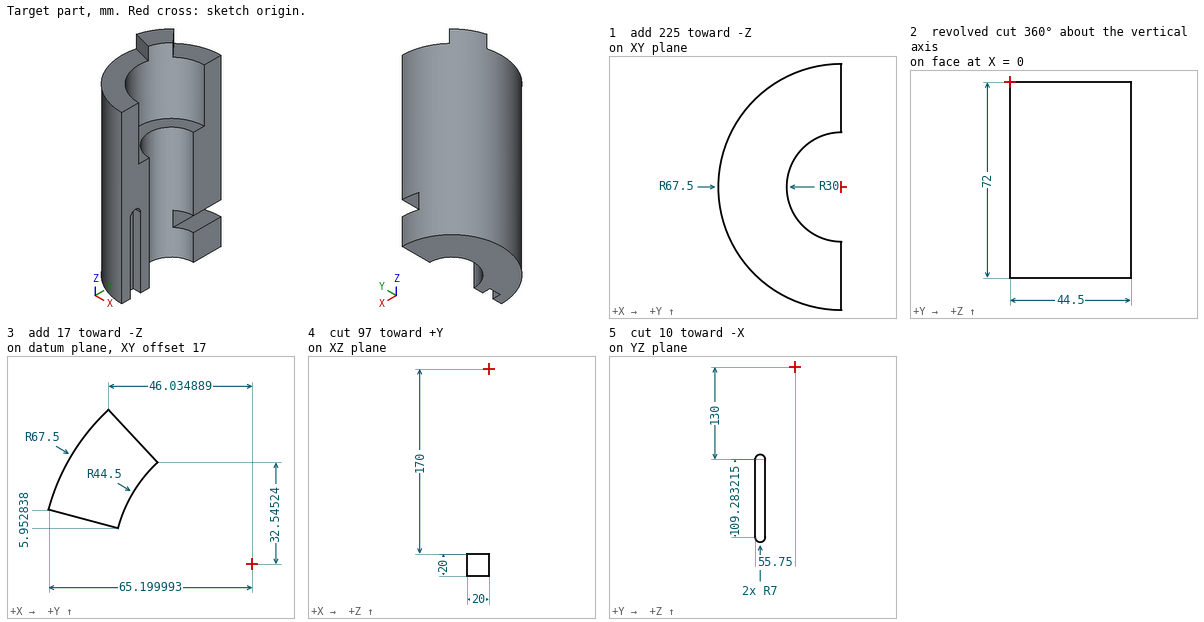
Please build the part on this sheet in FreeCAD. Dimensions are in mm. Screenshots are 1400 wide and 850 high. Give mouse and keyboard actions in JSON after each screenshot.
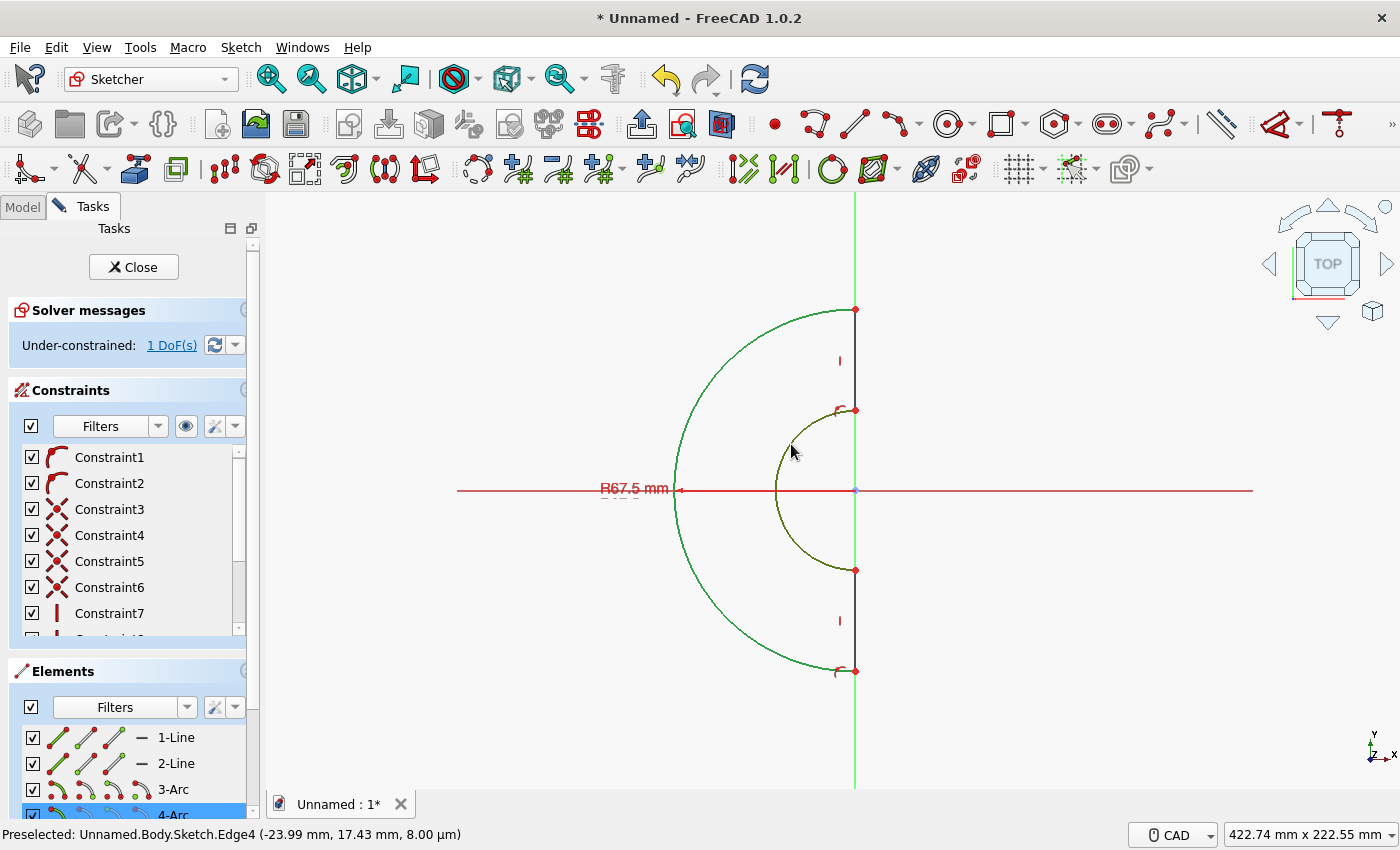
{"action": "key", "text": "k r"}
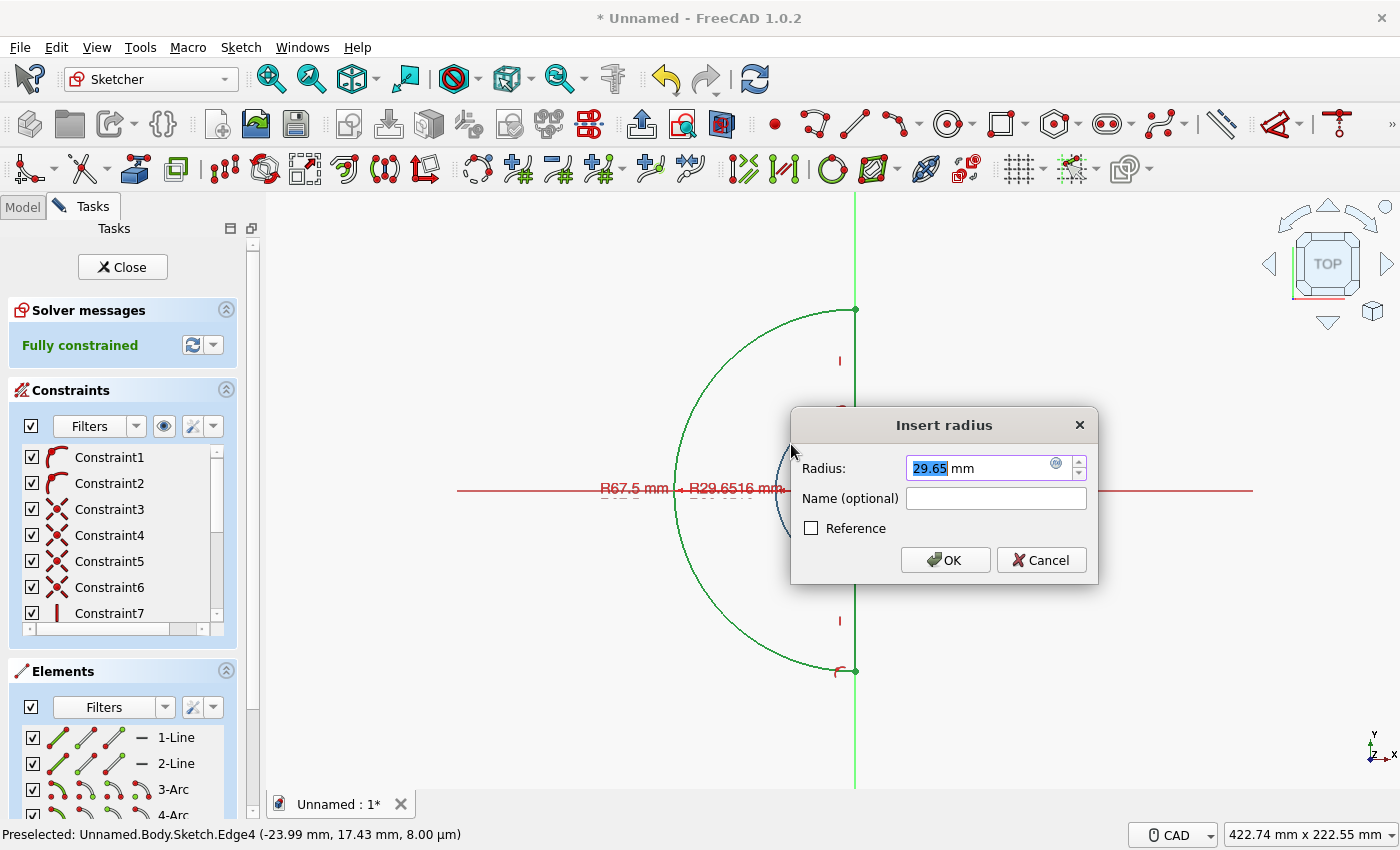
{"action": "type", "text": "30"}
{"action": "key", "text": "Return"}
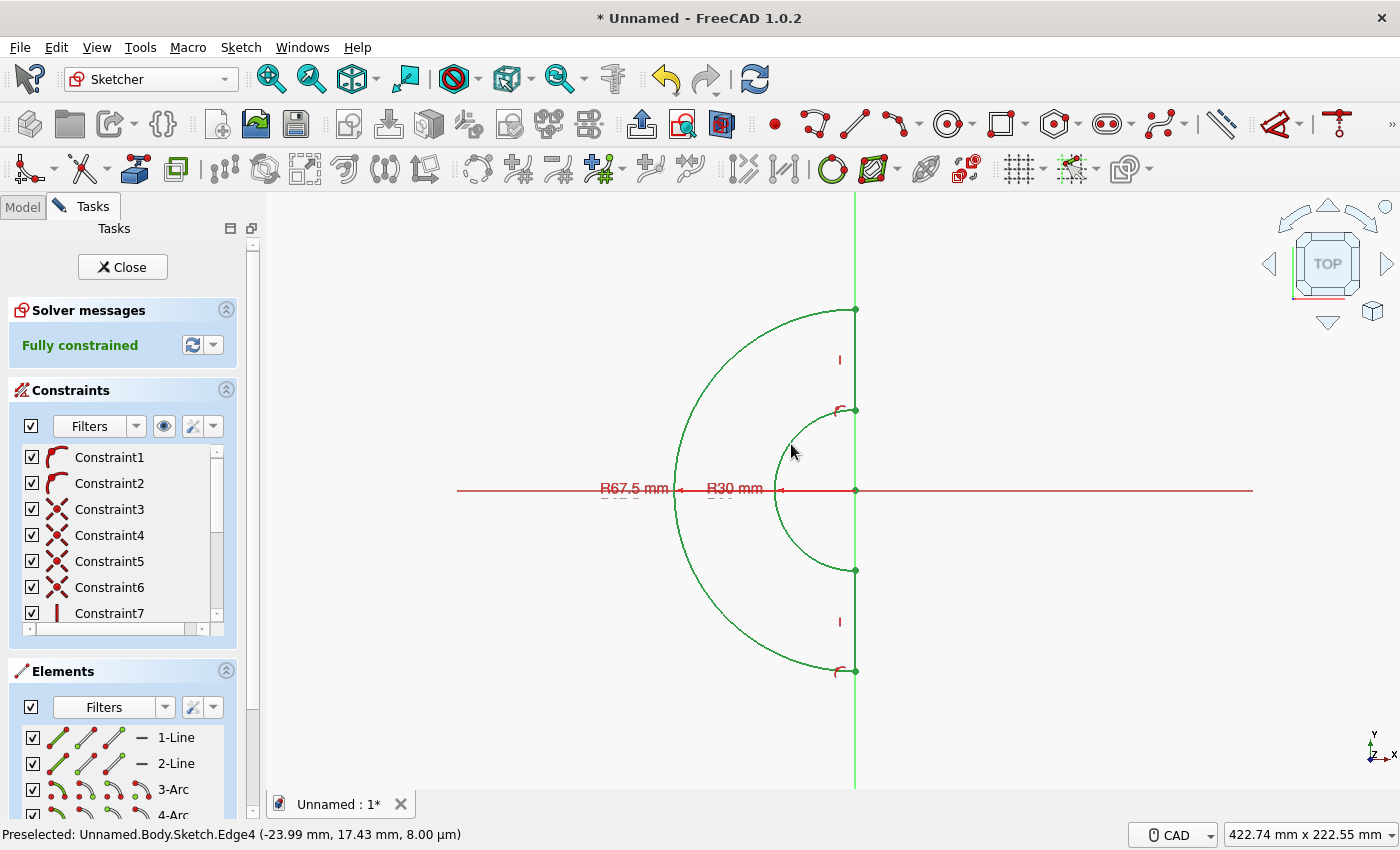
{"action": "left_click", "coordinate": [123, 267]}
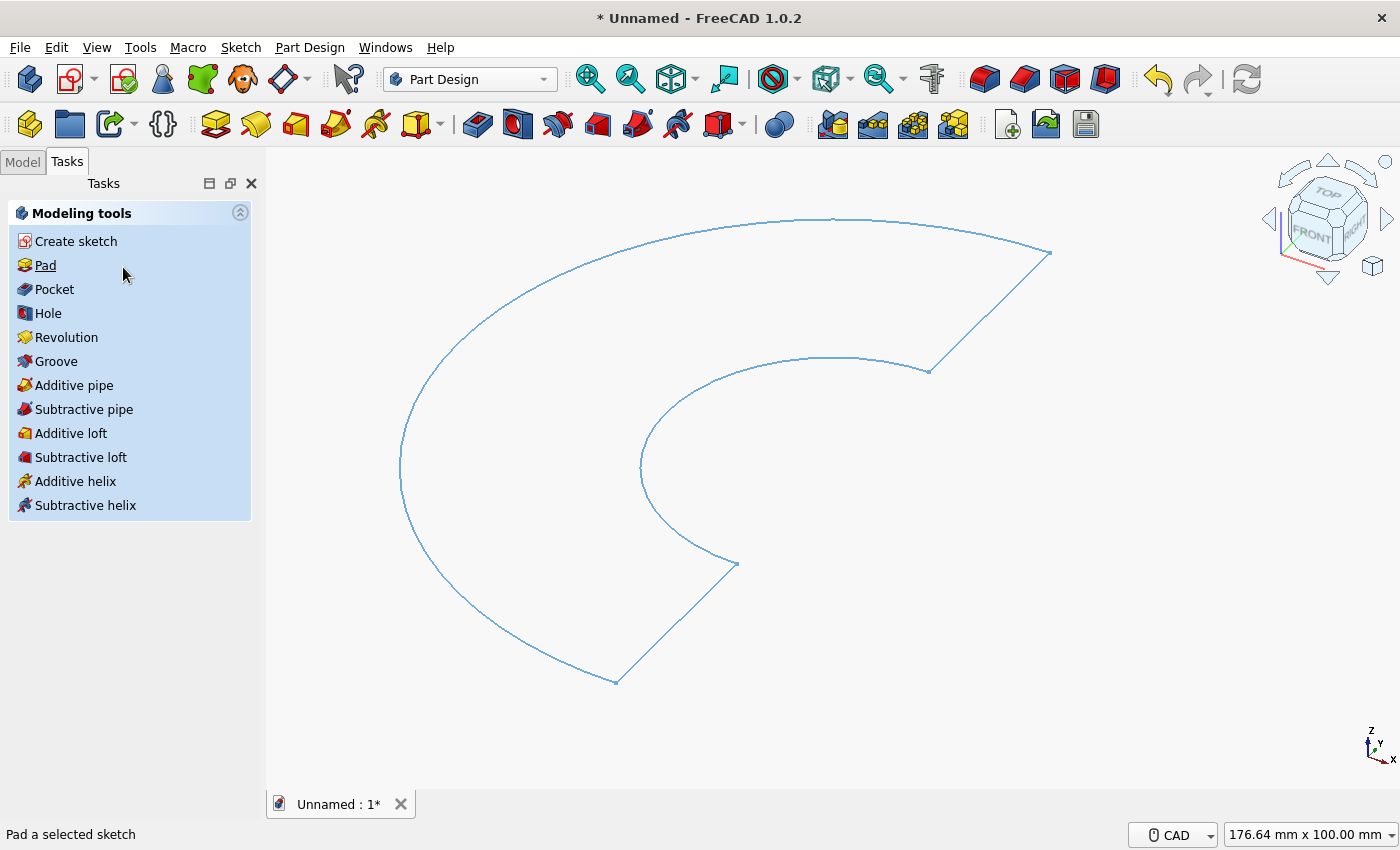
{"action": "left_click", "coordinate": [216, 124]}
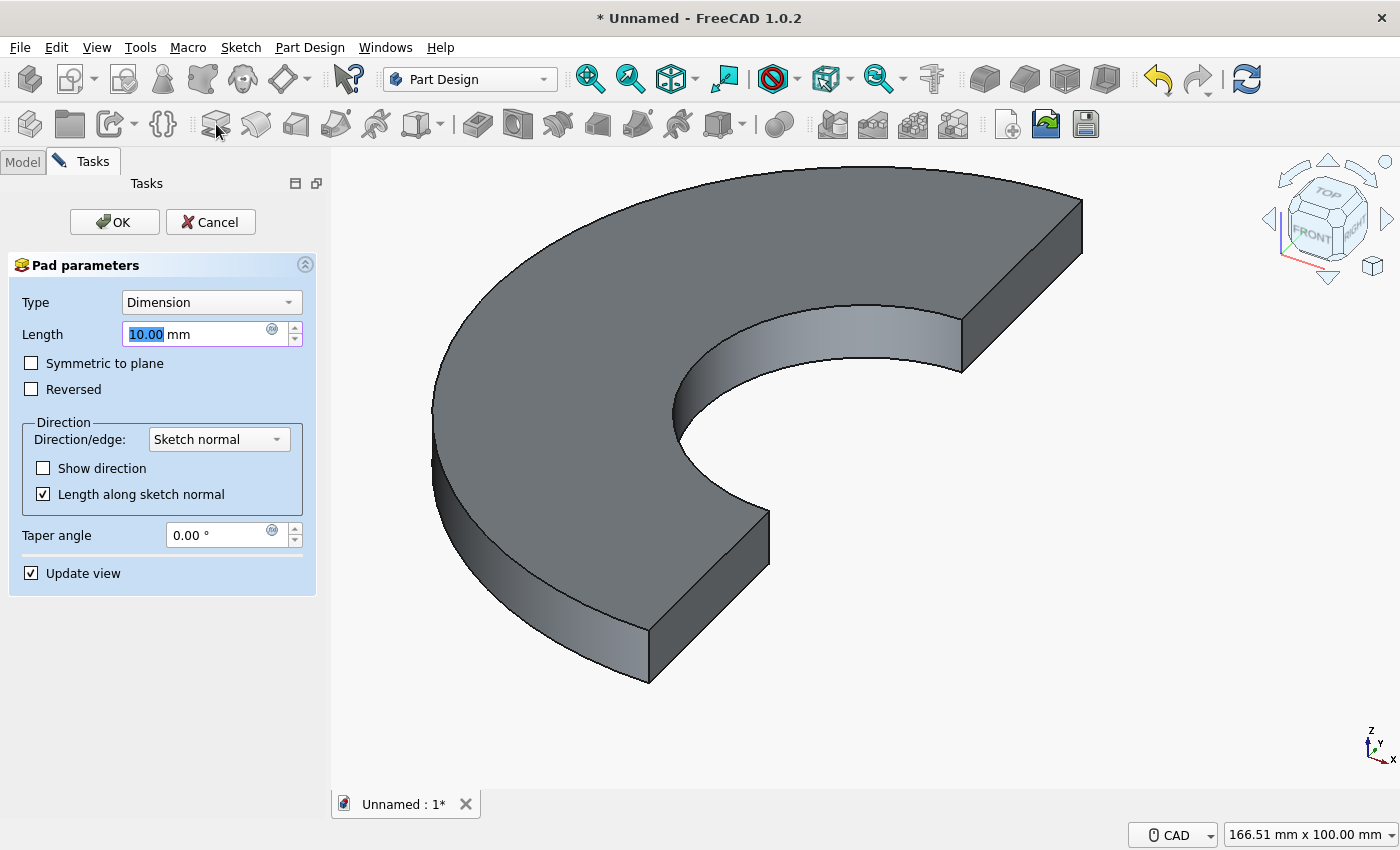
{"action": "type", "text": "225"}
{"action": "key", "text": "Tab"}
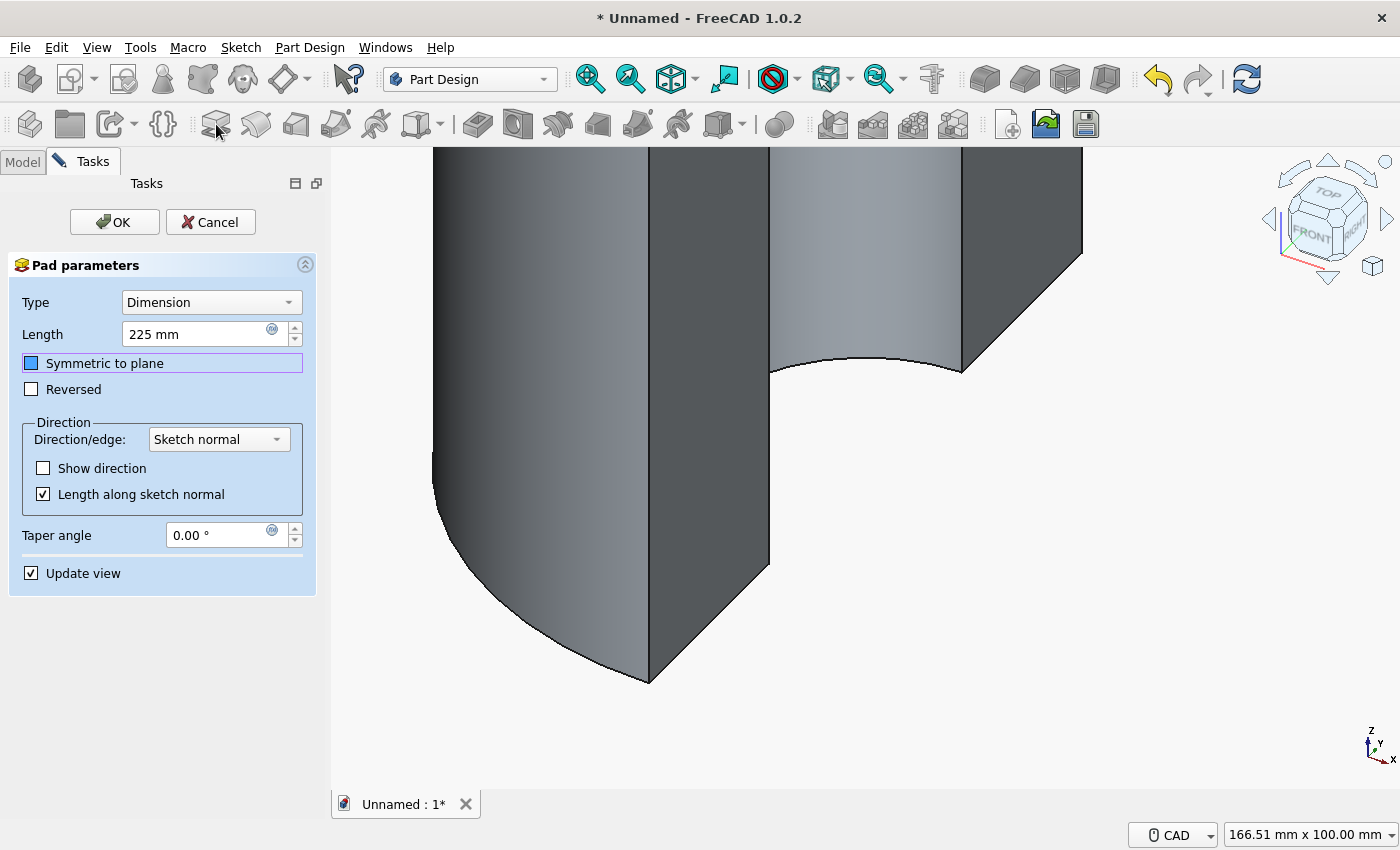
{"action": "left_click", "coordinate": [30, 389]}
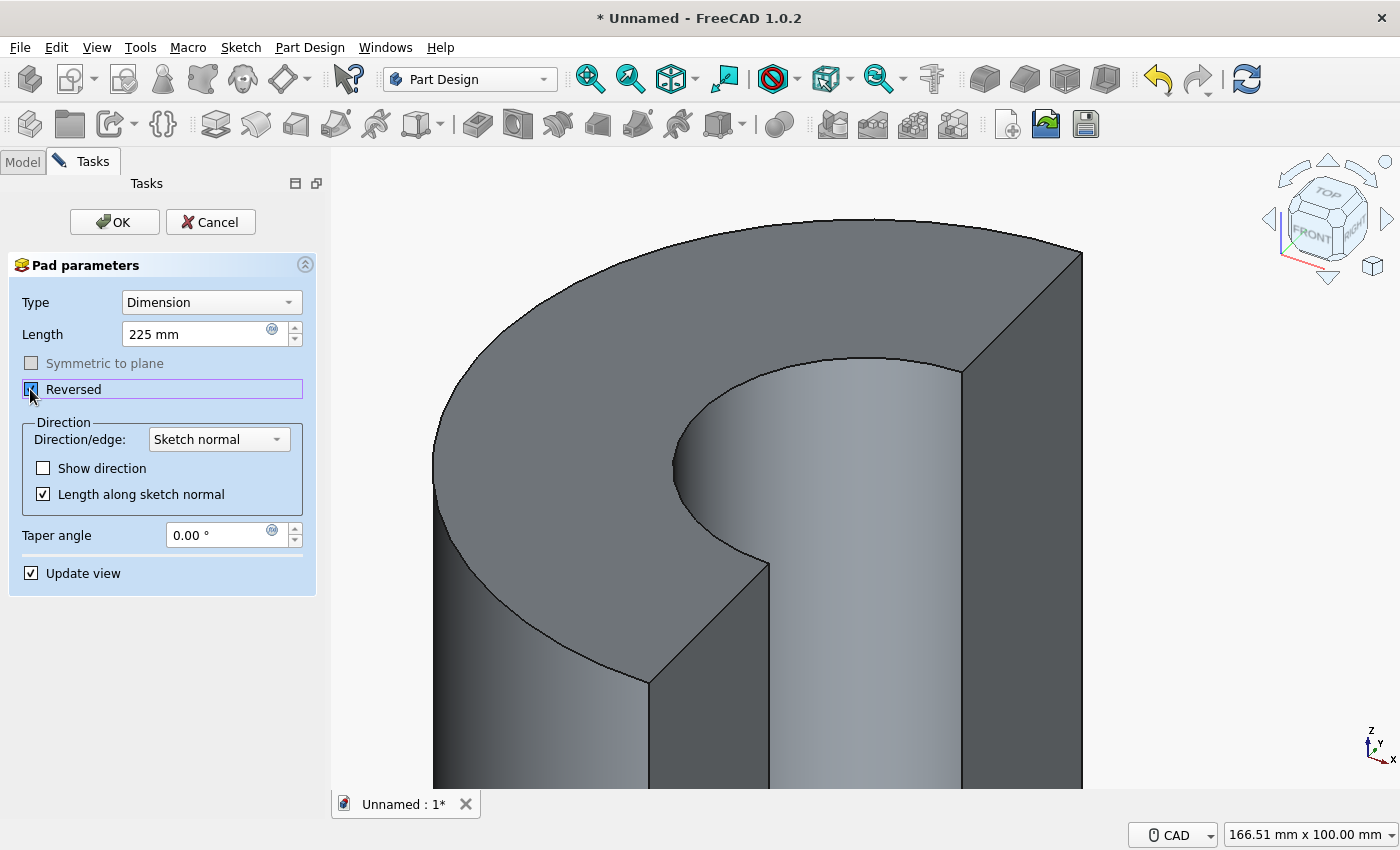
{"action": "left_click", "coordinate": [115, 222]}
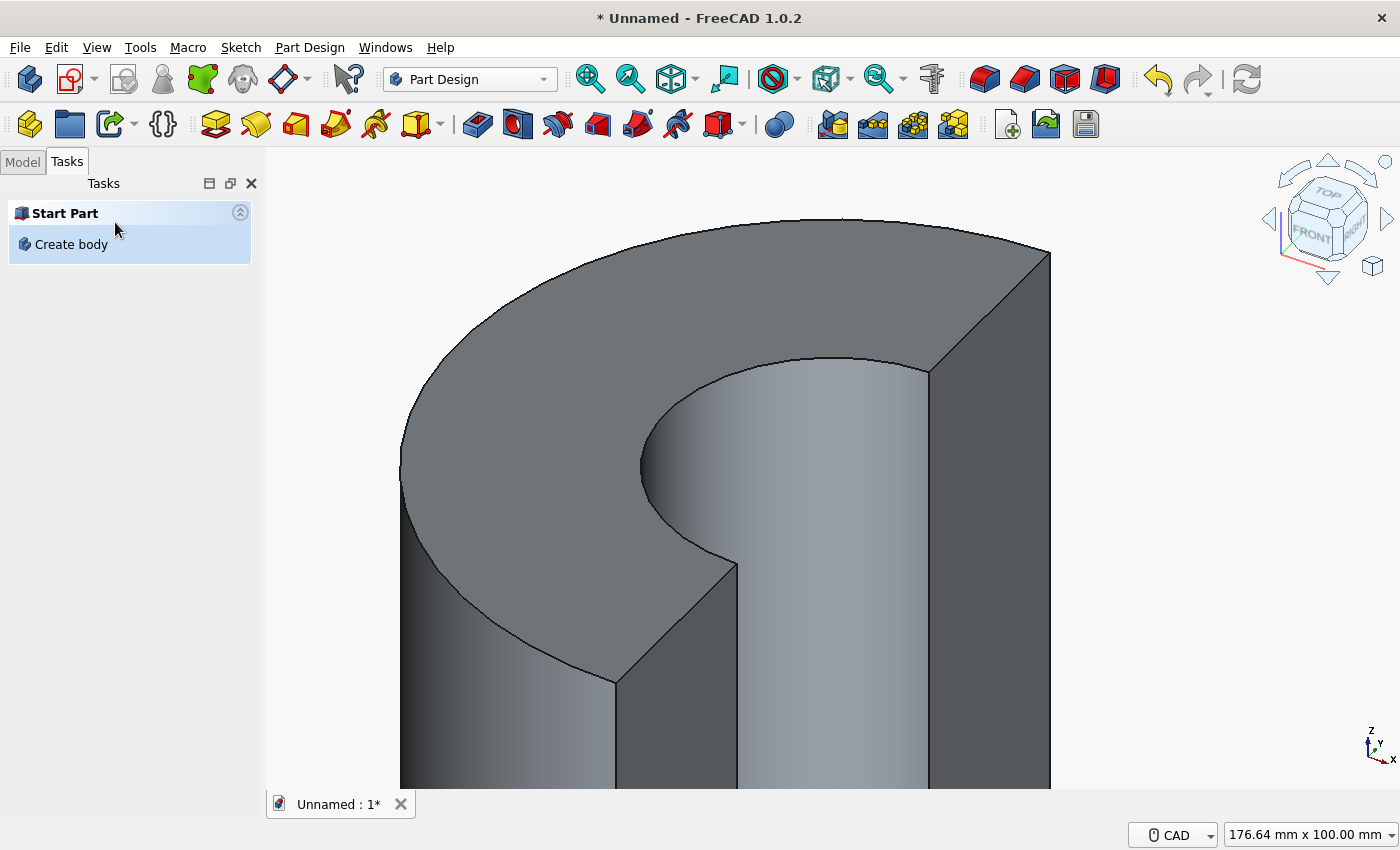
{"action": "left_click", "coordinate": [592, 80]}